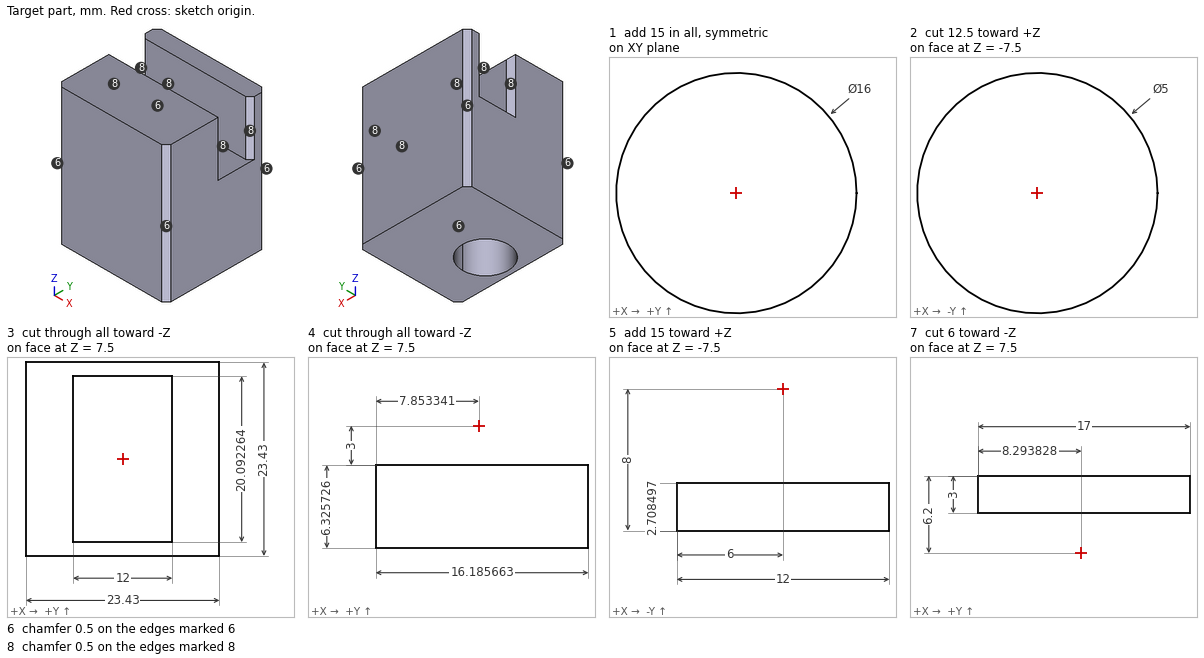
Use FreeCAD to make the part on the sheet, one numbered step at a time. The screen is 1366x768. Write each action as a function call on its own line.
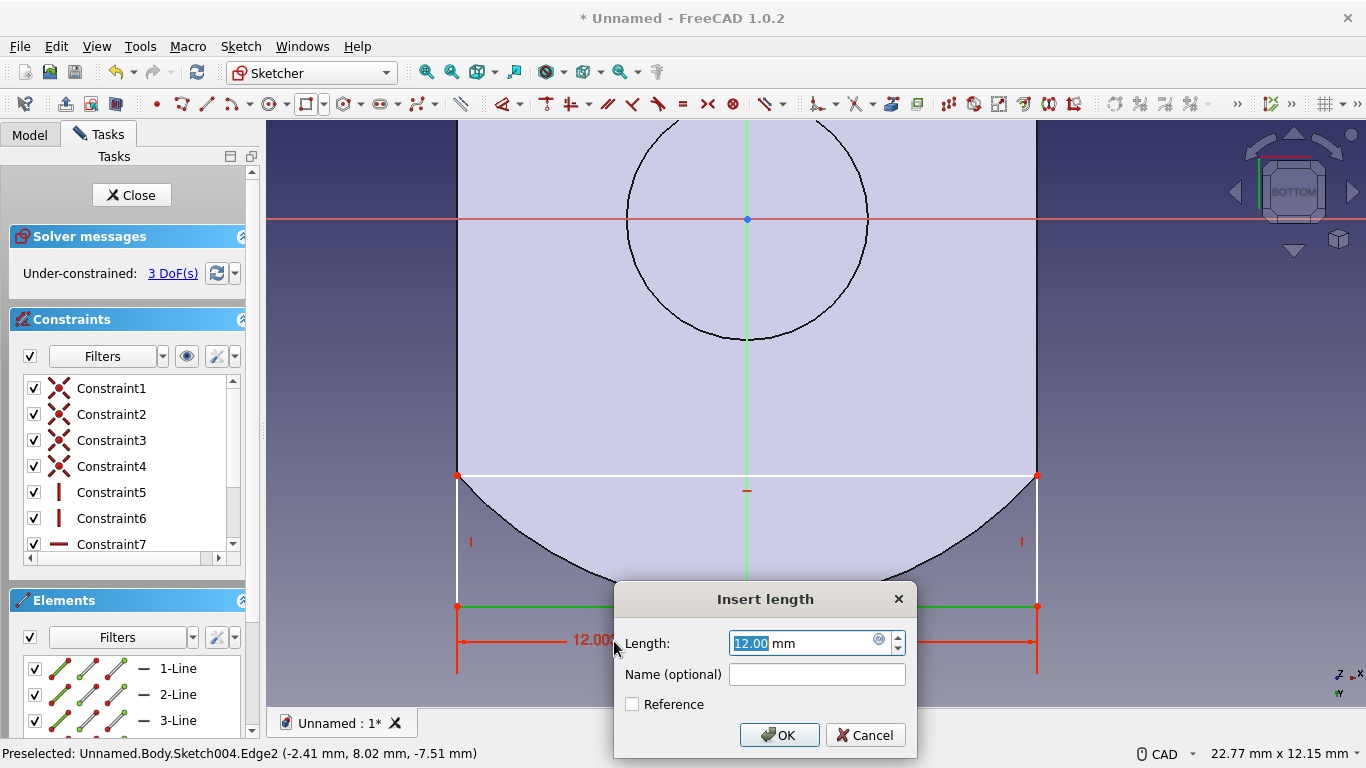
text(12)
key(Return)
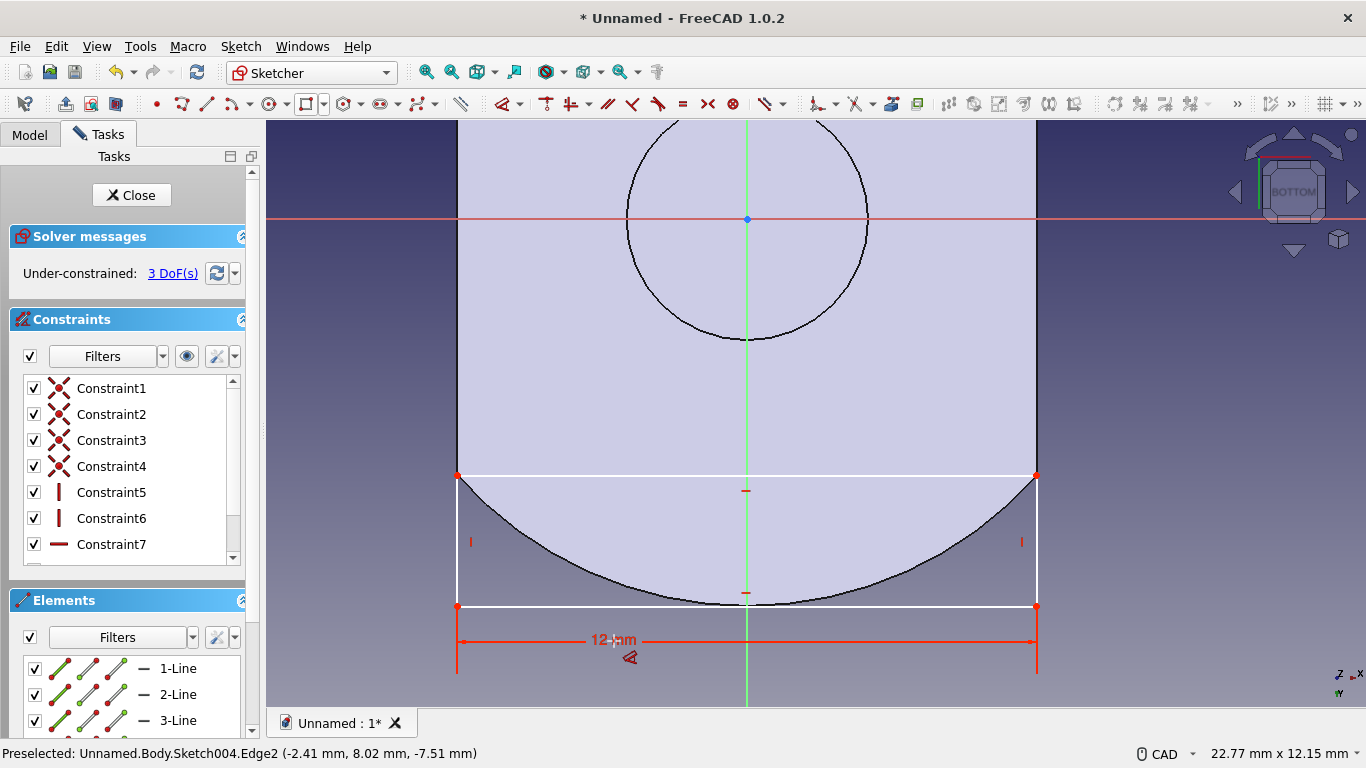
click(457, 476)
click(602, 185)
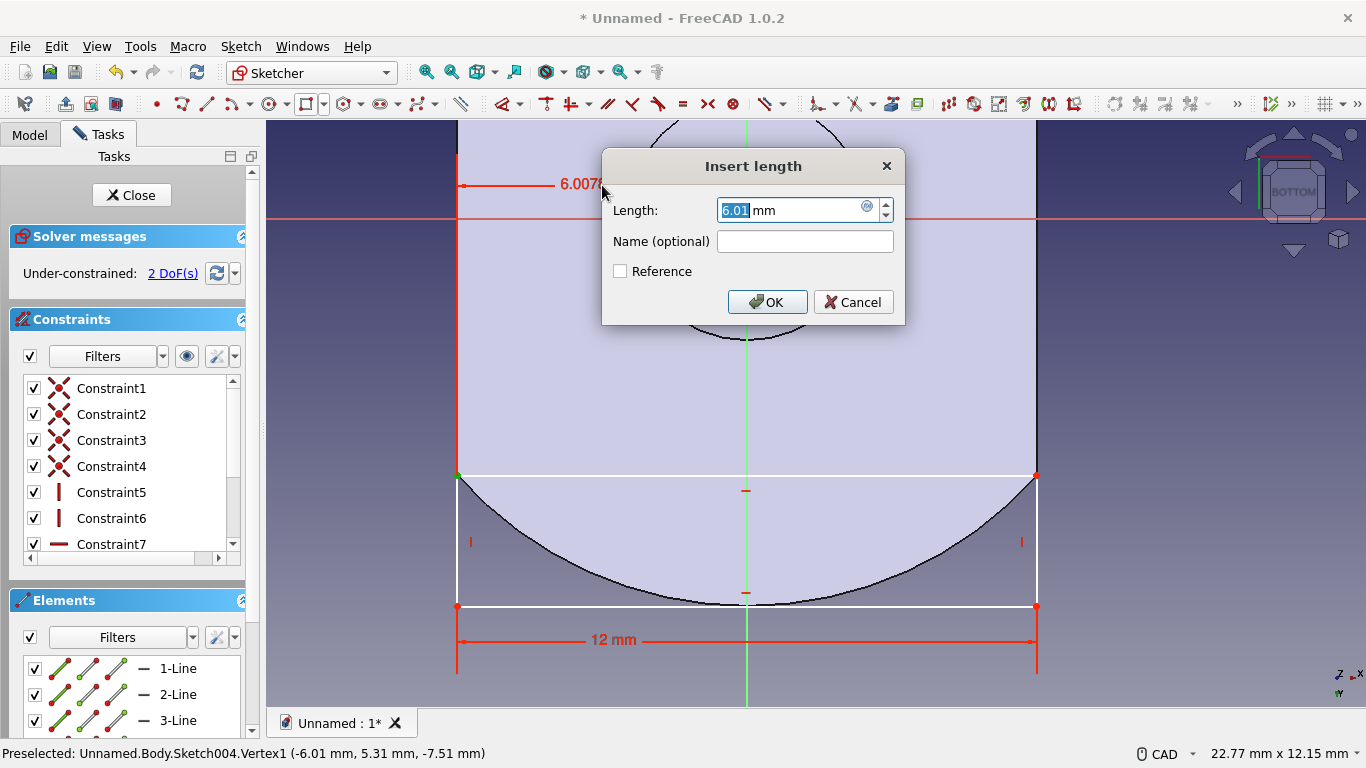
text(6)
key(Return)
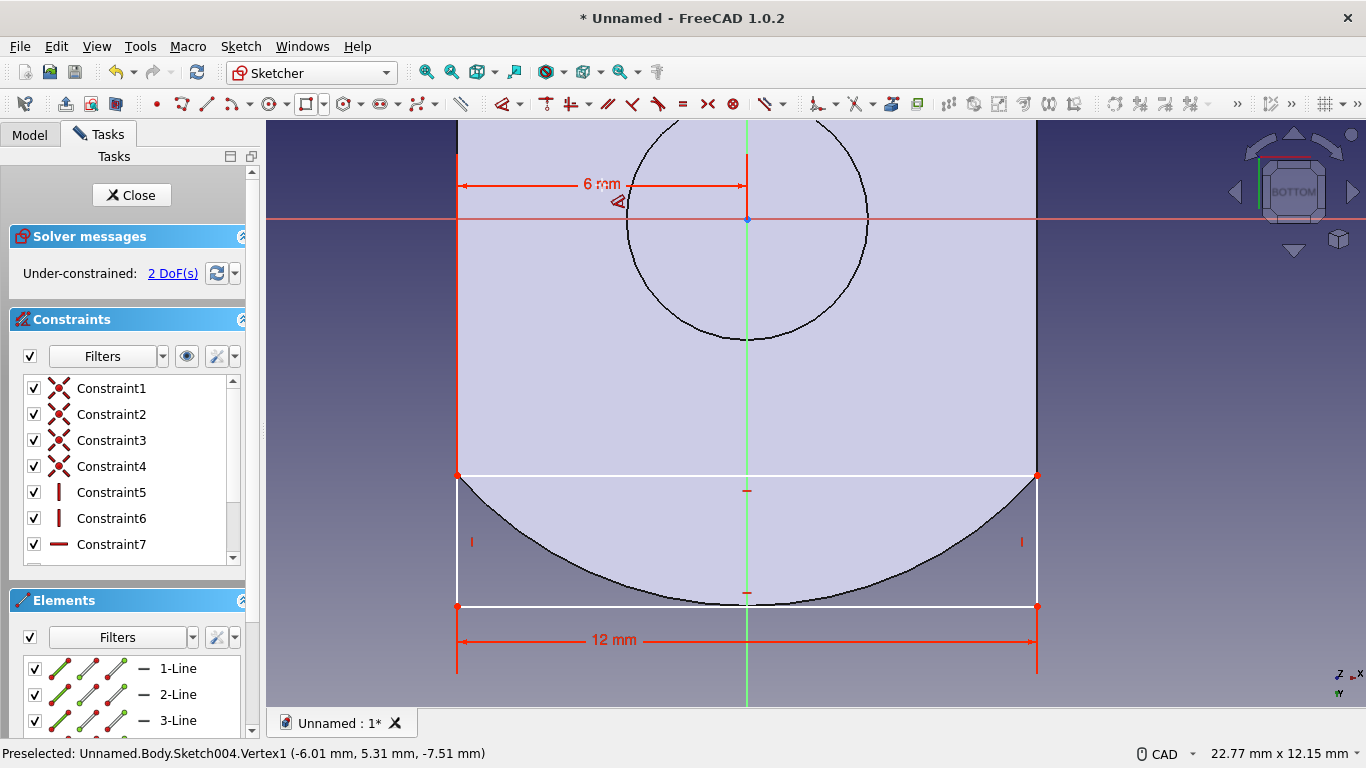
click(457, 607)
click(423, 413)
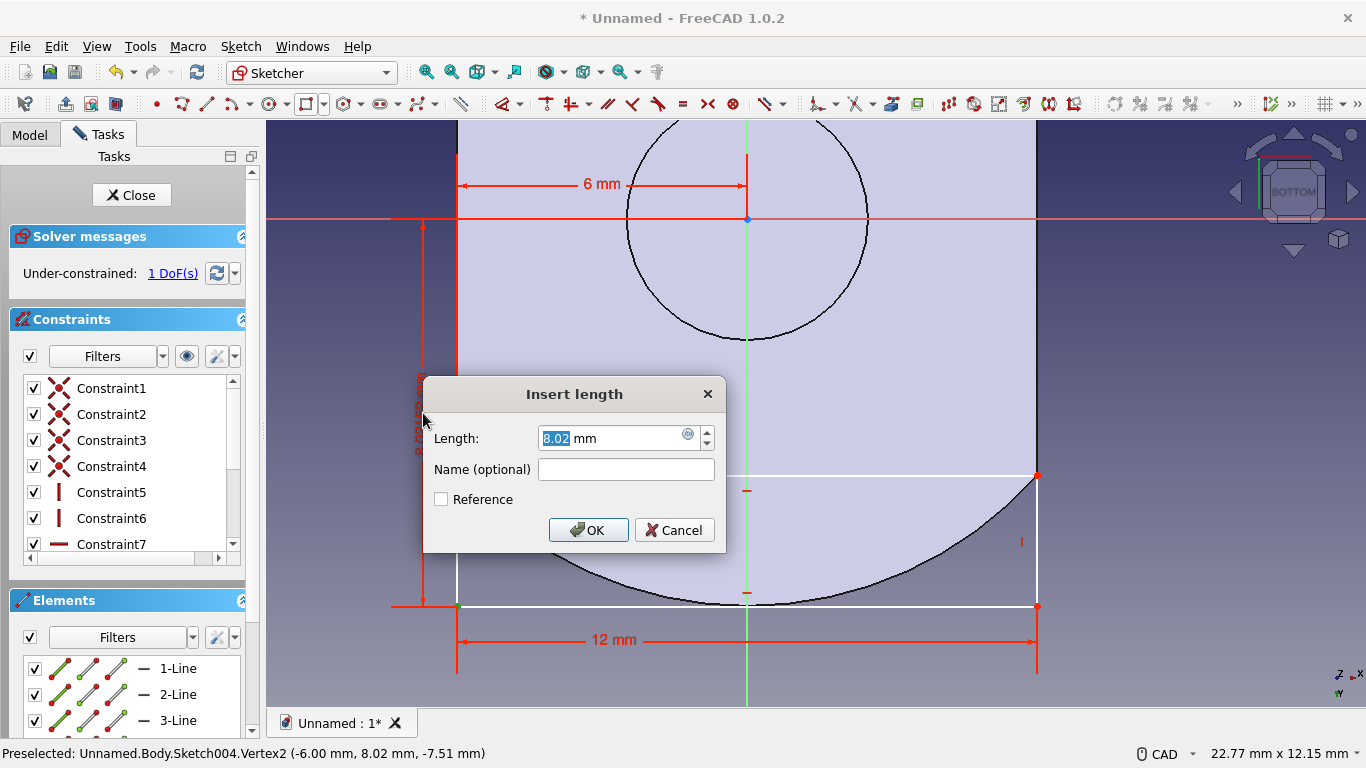
text(8)
key(Return)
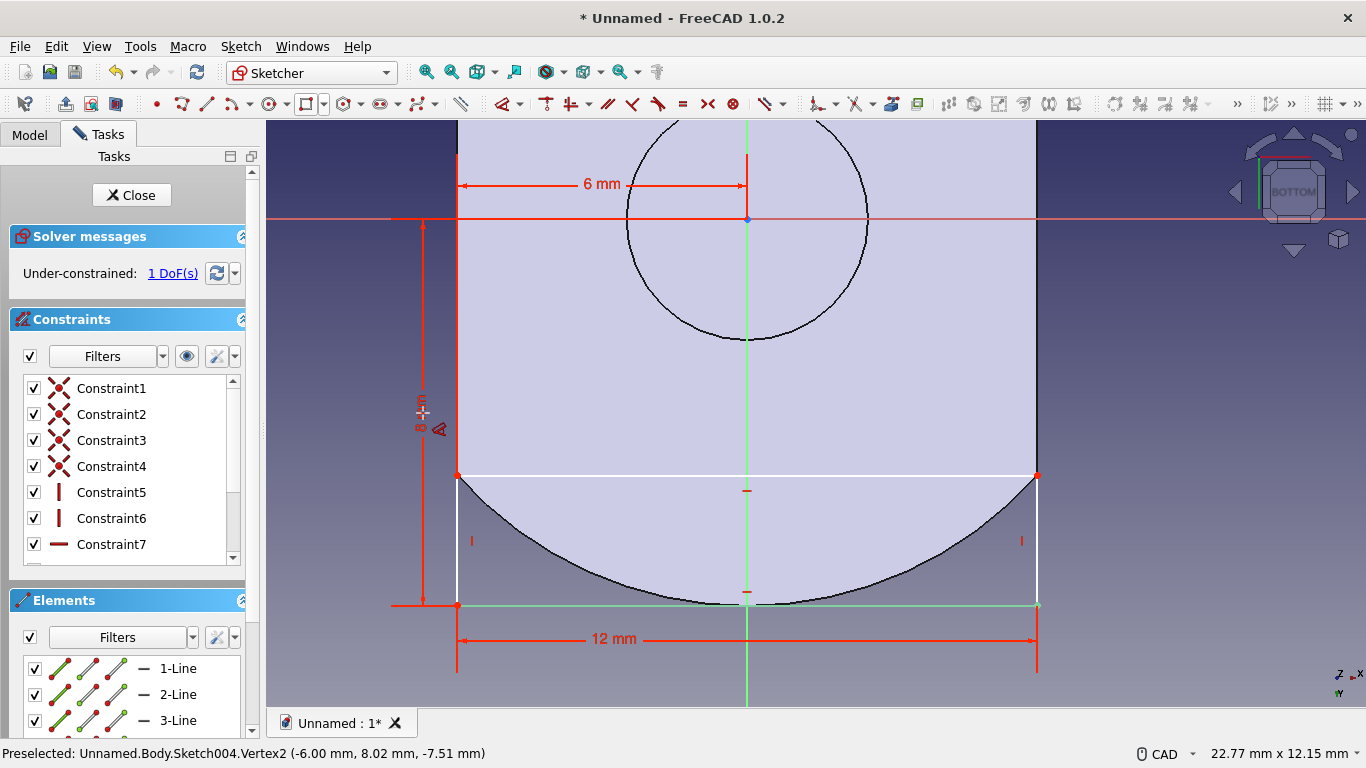
click(457, 515)
click(423, 541)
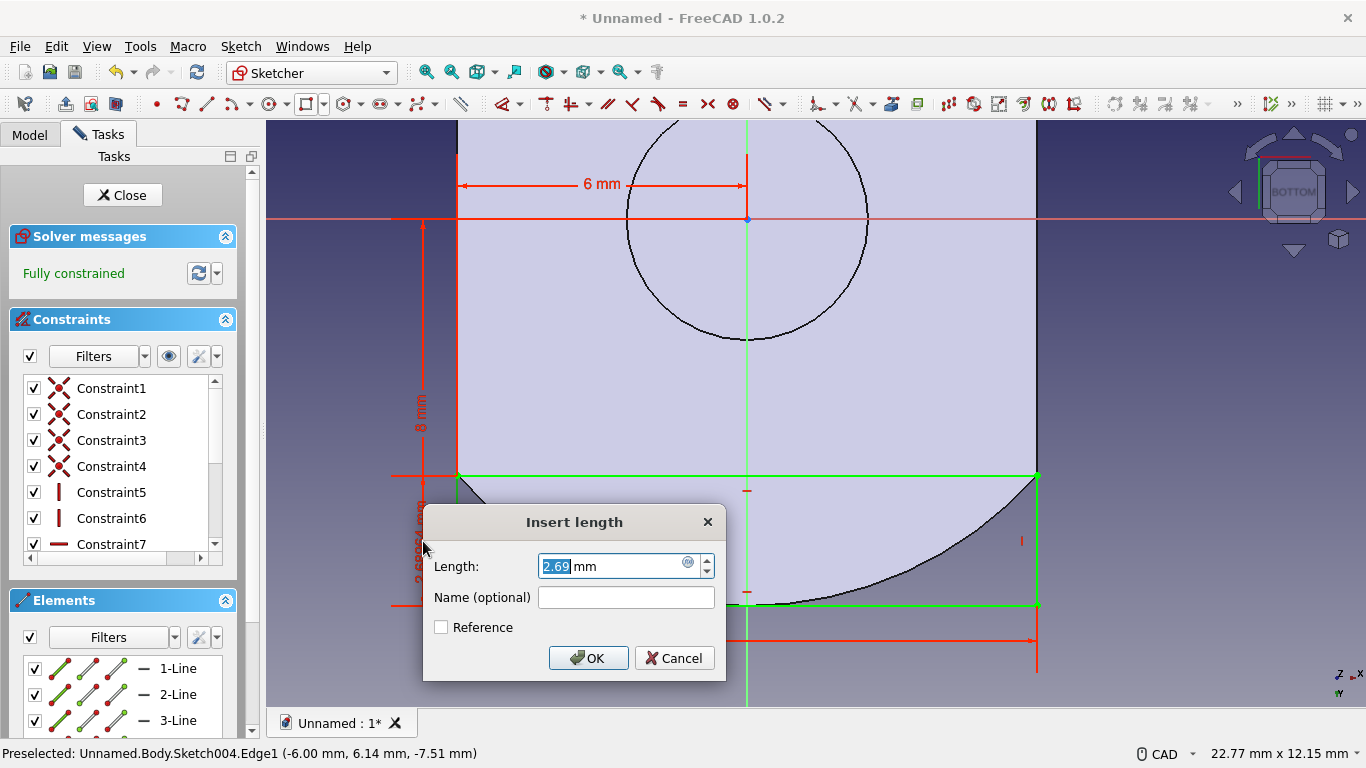
text(2.708497)
key(Return)
key(Escape)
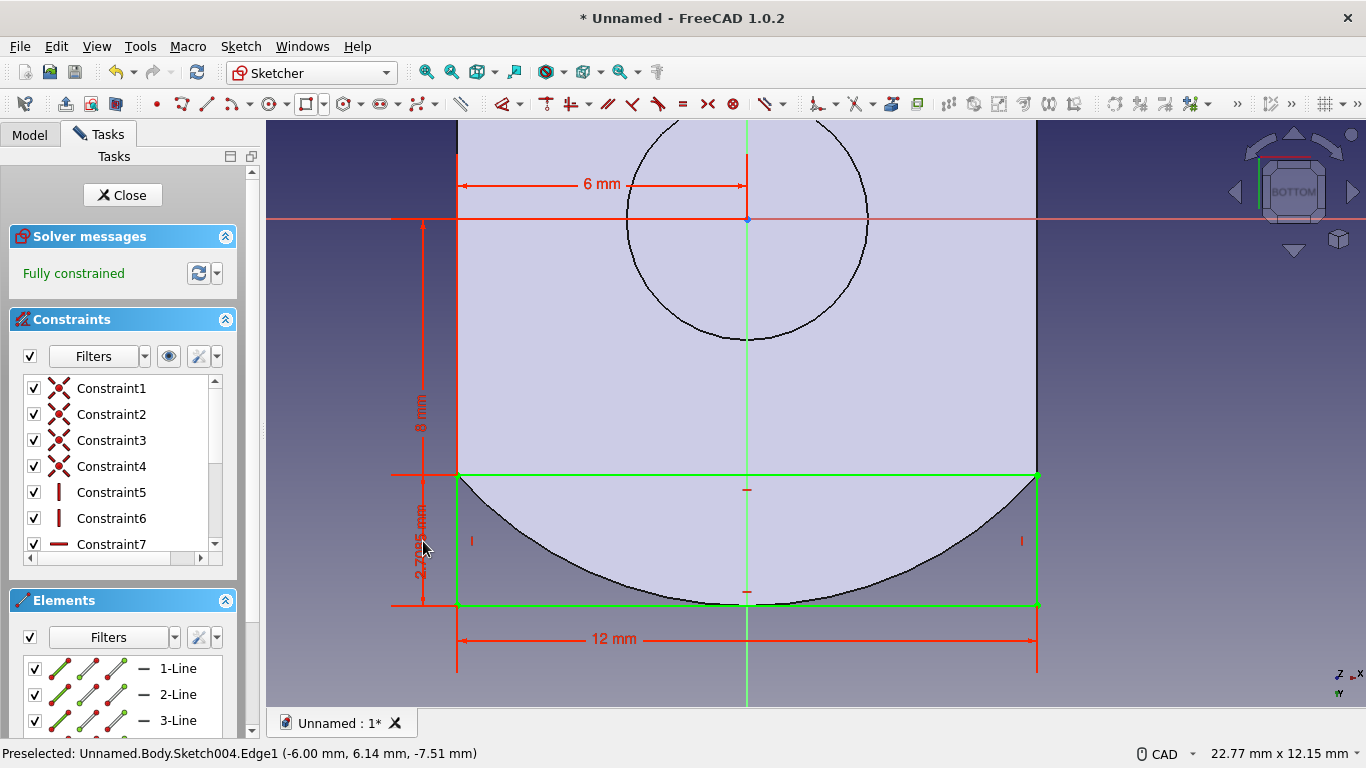
click(123, 195)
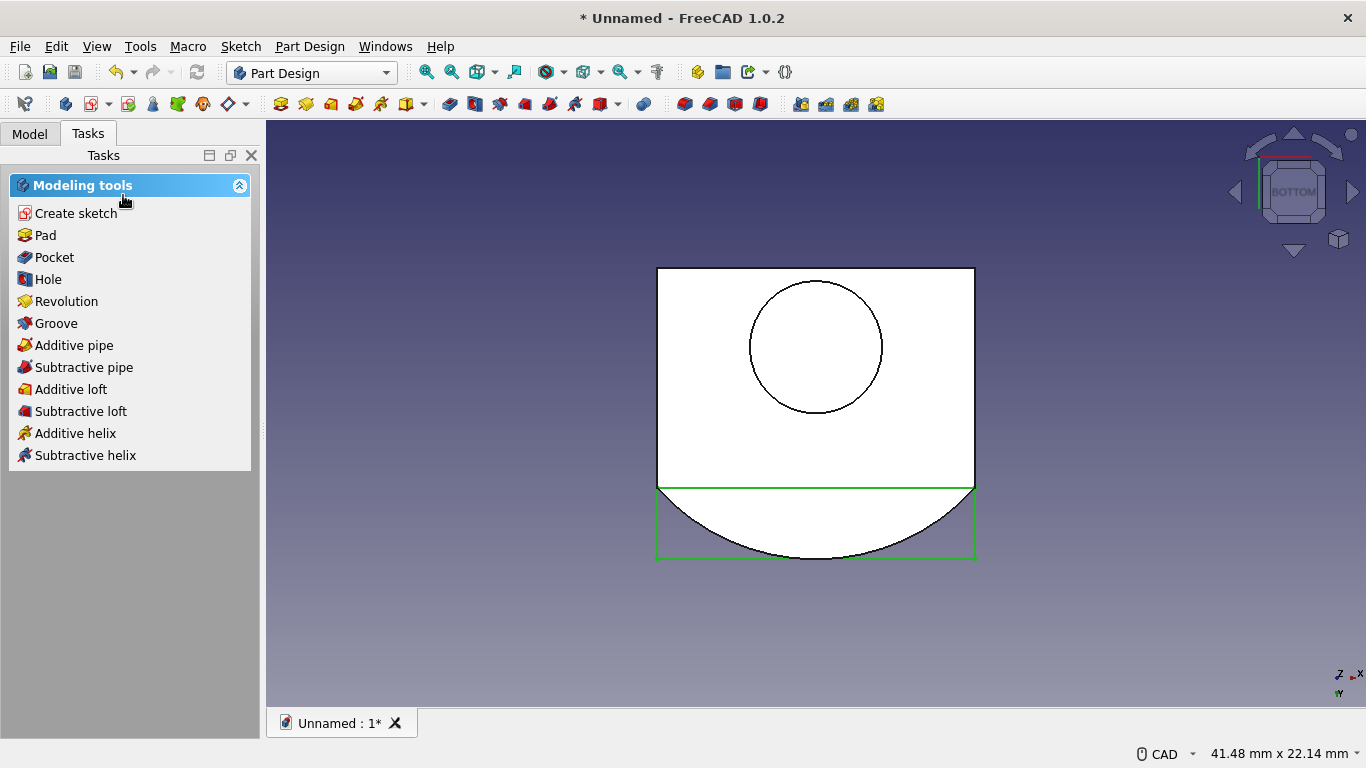
click(281, 104)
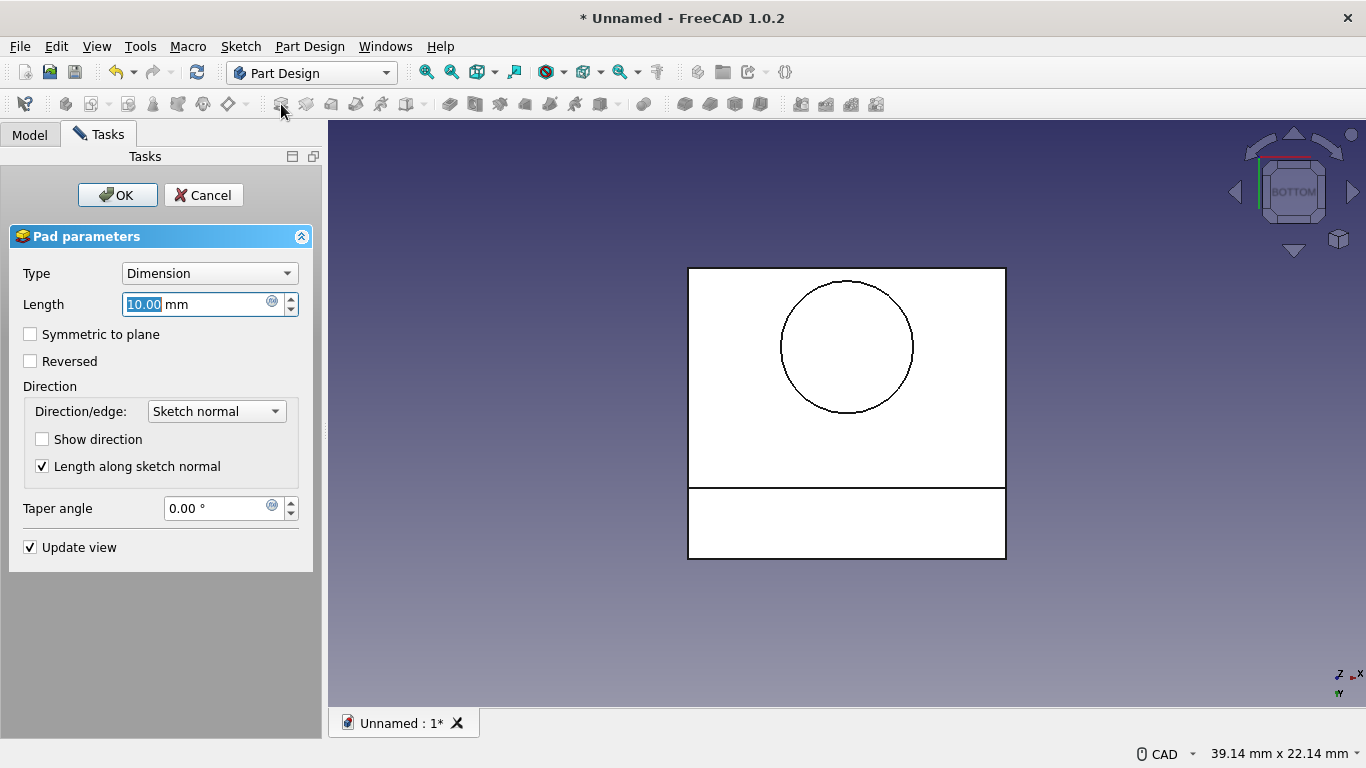
text(15)
key(Tab)